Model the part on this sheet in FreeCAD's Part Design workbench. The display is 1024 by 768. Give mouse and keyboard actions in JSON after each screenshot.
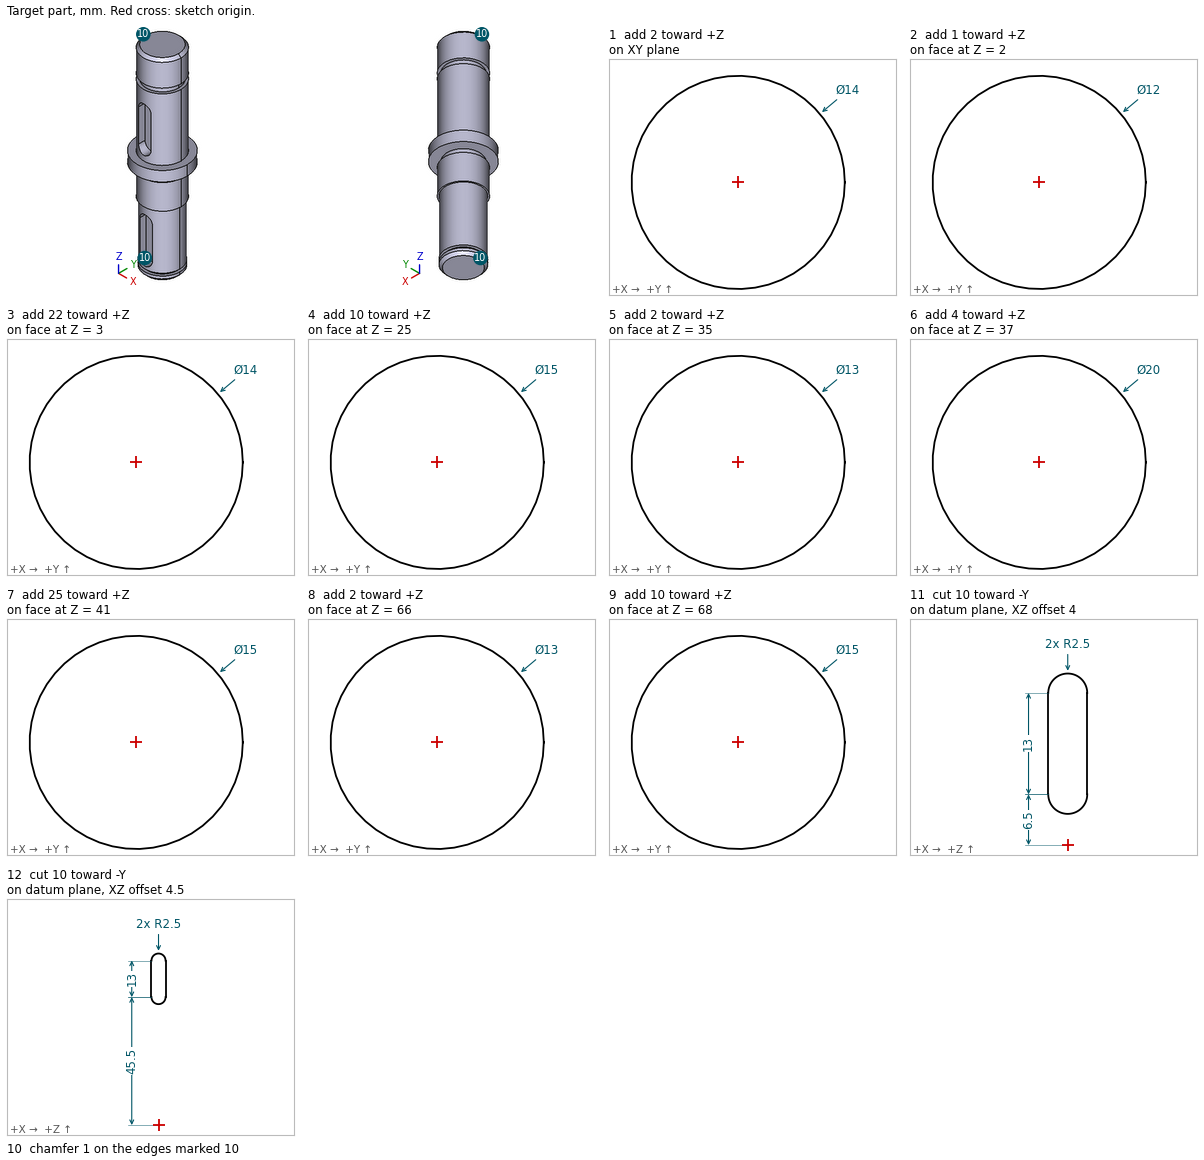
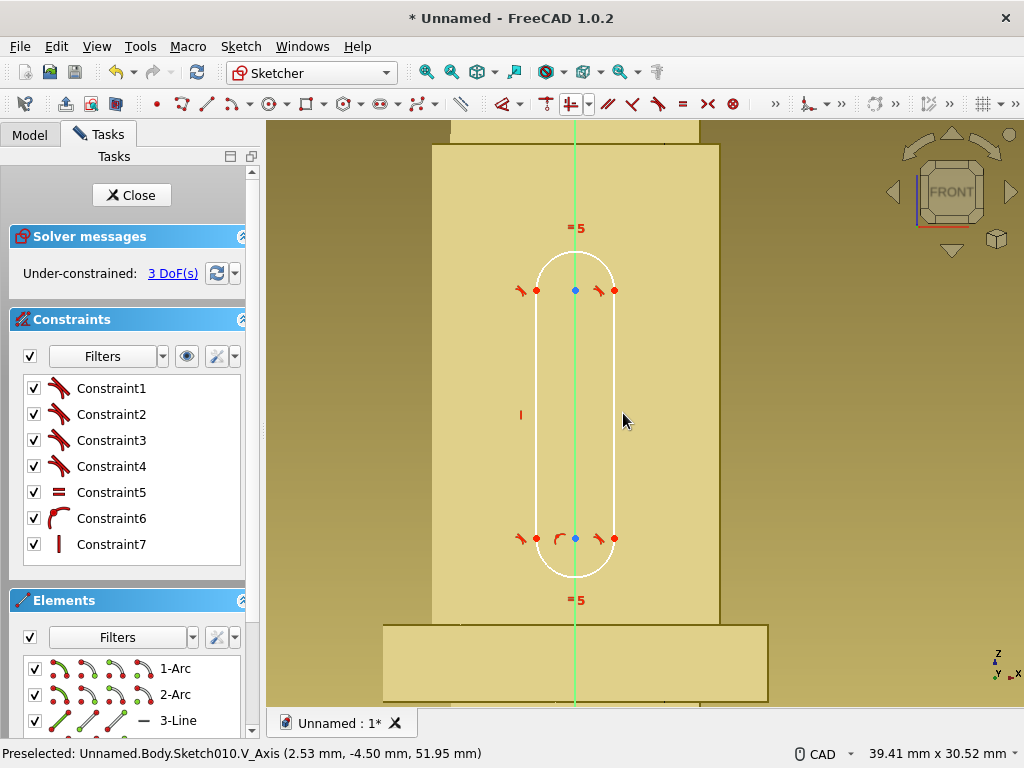
{"action": "left_click", "coordinate": [502, 104]}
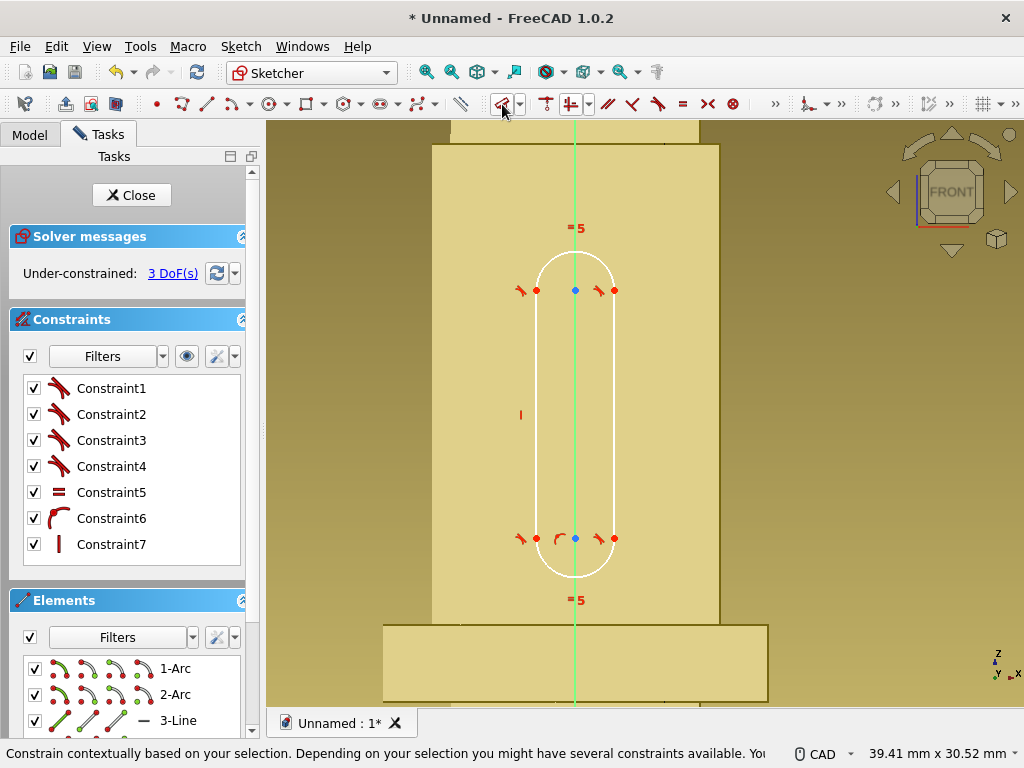
{"action": "left_click", "coordinate": [552, 570]}
{"action": "left_click", "coordinate": [533, 596]}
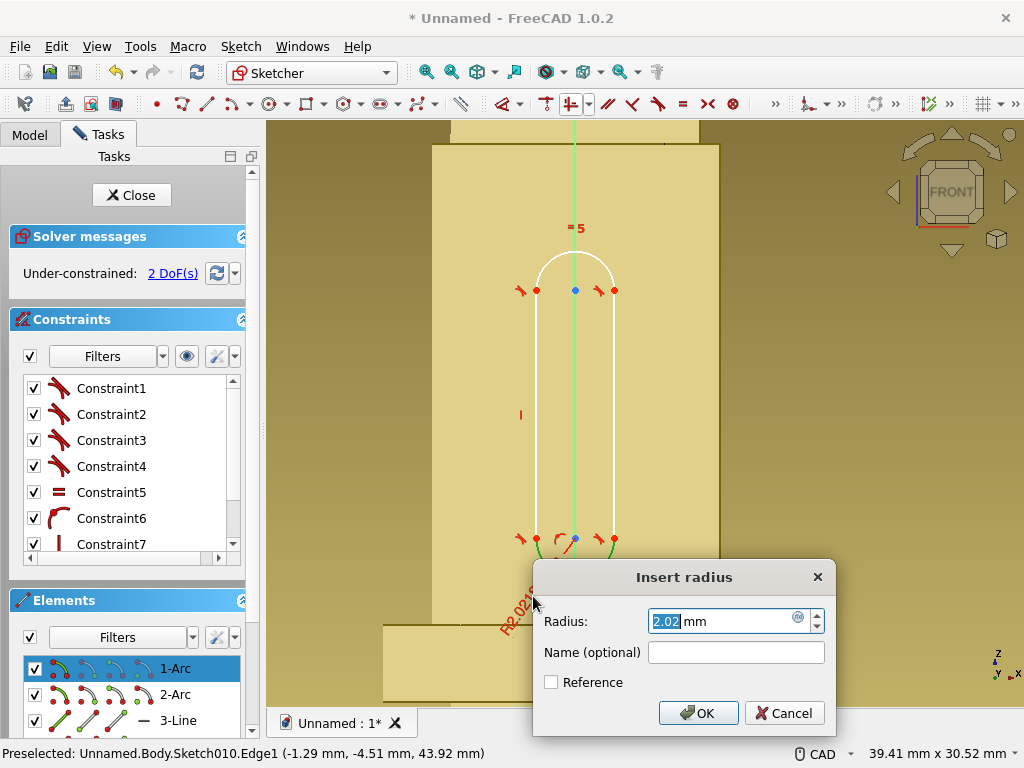
{"action": "type", "text": "2.5"}
{"action": "key", "text": "Return"}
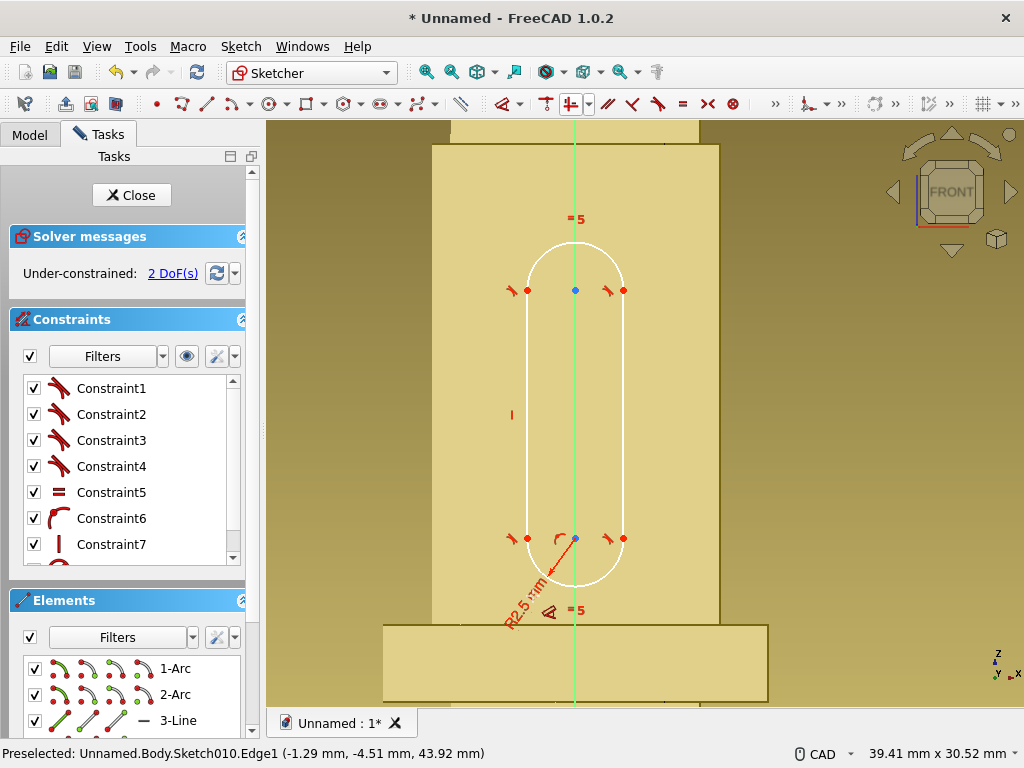
{"action": "left_click", "coordinate": [527, 464]}
{"action": "left_click", "coordinate": [493, 415]}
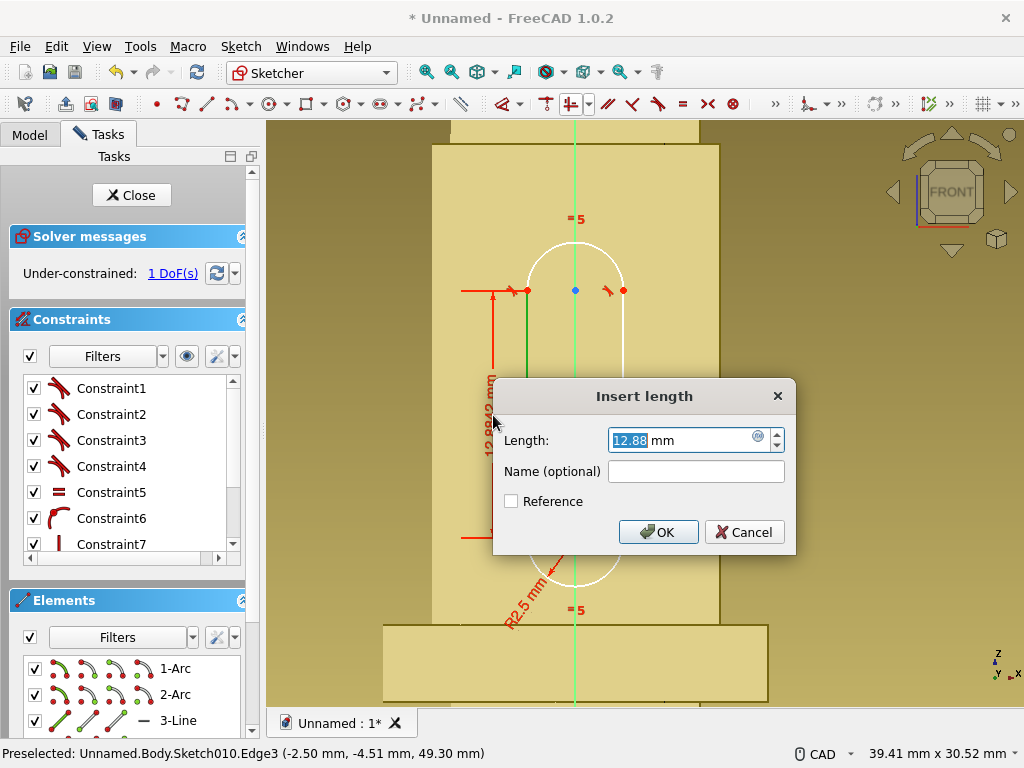
{"action": "type", "text": "13"}
{"action": "key", "text": "Return"}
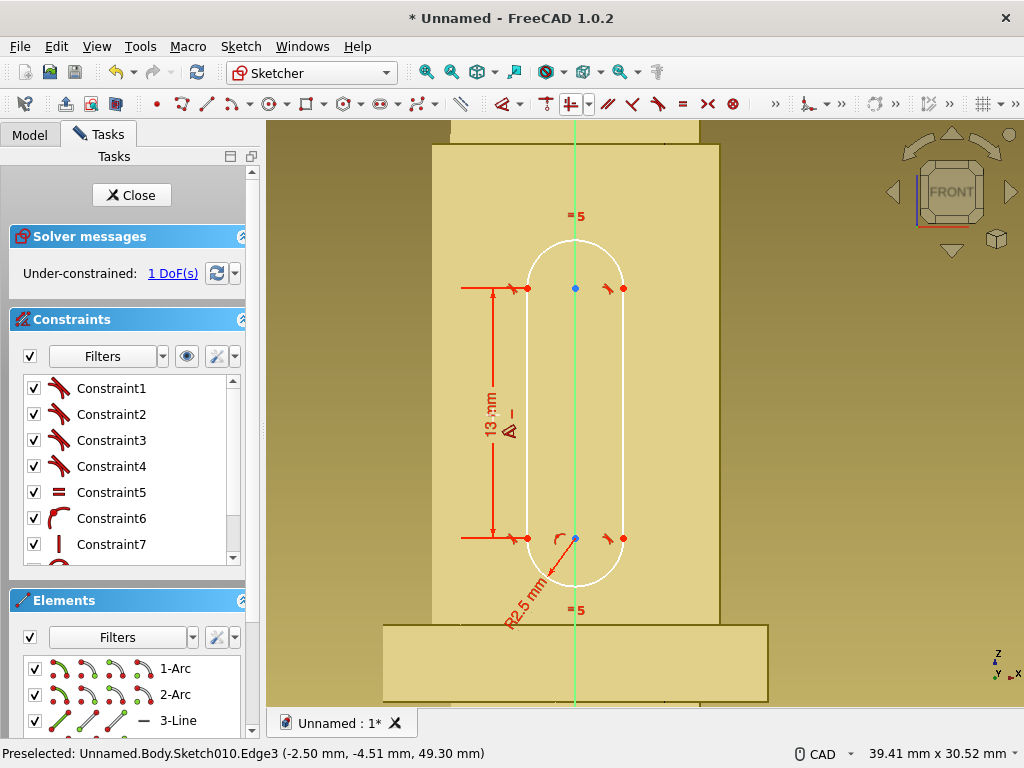
{"action": "left_click", "coordinate": [527, 538]}
{"action": "left_click", "coordinate": [493, 641]}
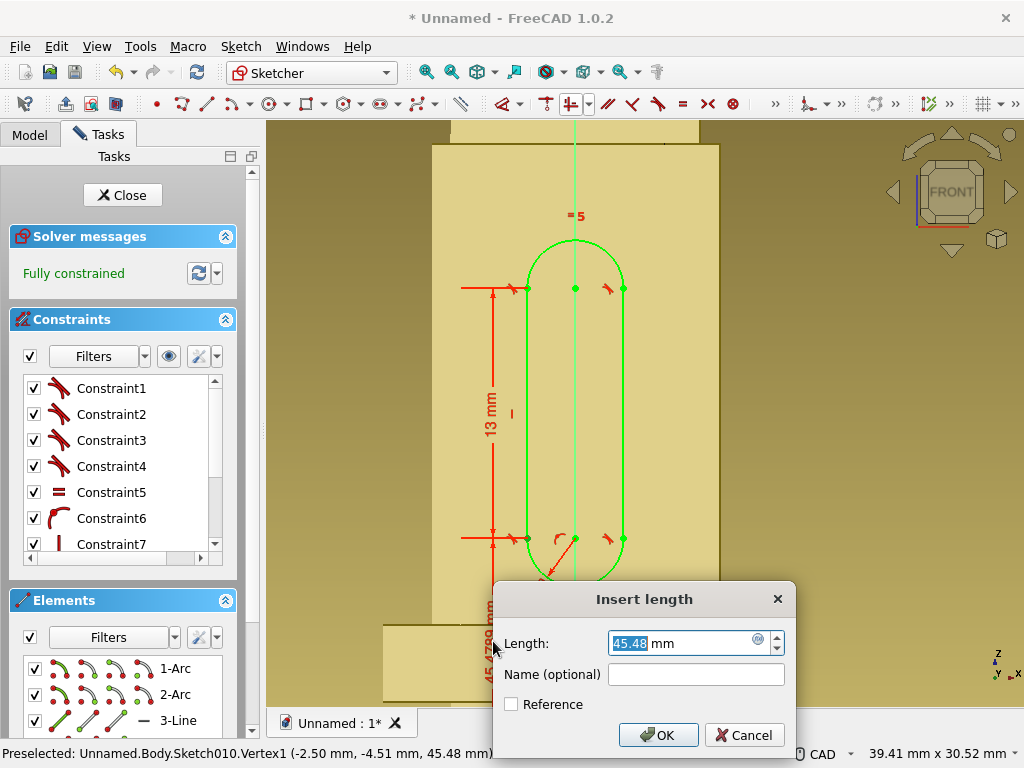
{"action": "type", "text": "45.5"}
{"action": "key", "text": "Return"}
{"action": "key", "text": "Escape"}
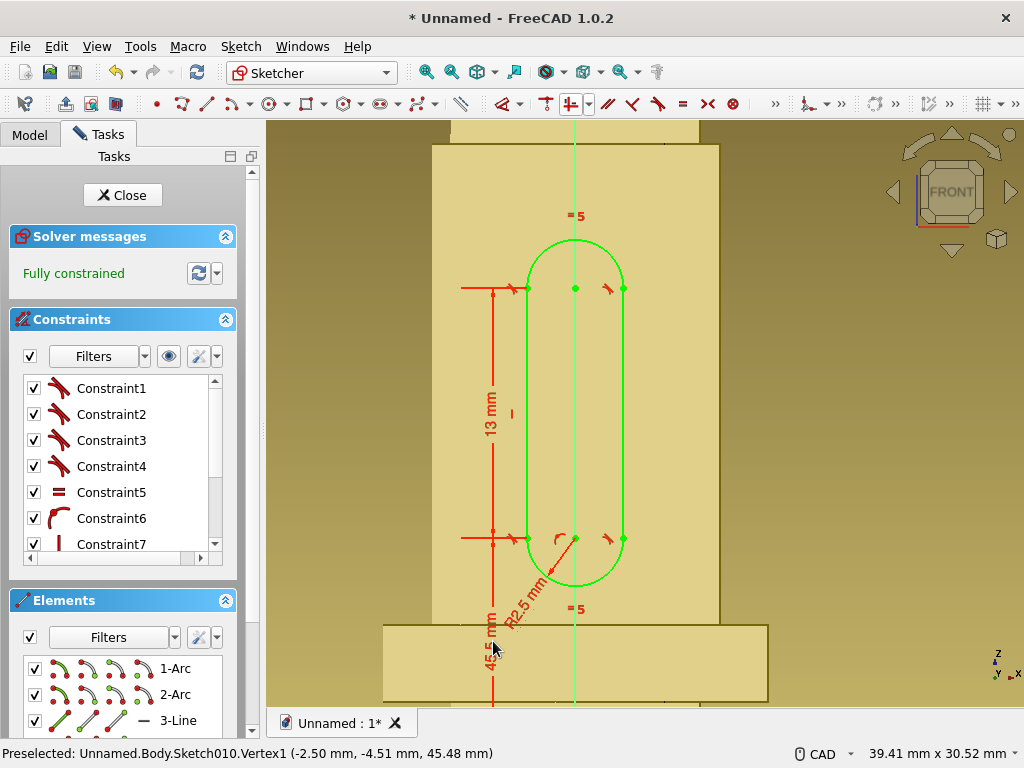
{"action": "left_click", "coordinate": [123, 195]}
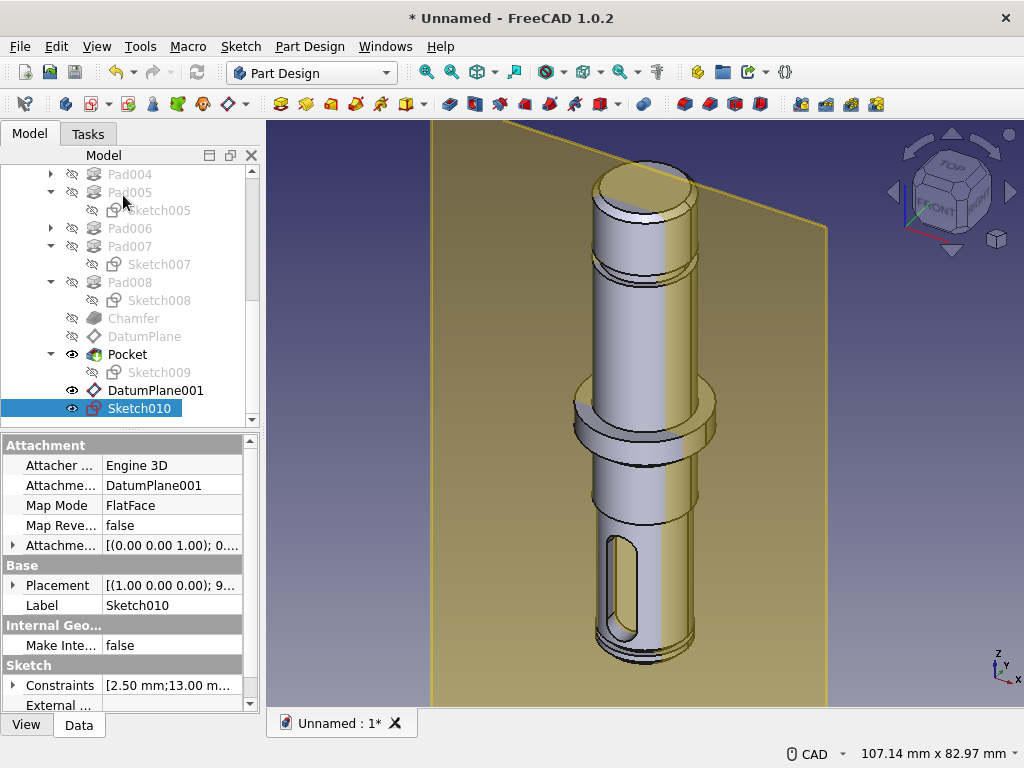
{"action": "left_click", "coordinate": [450, 104]}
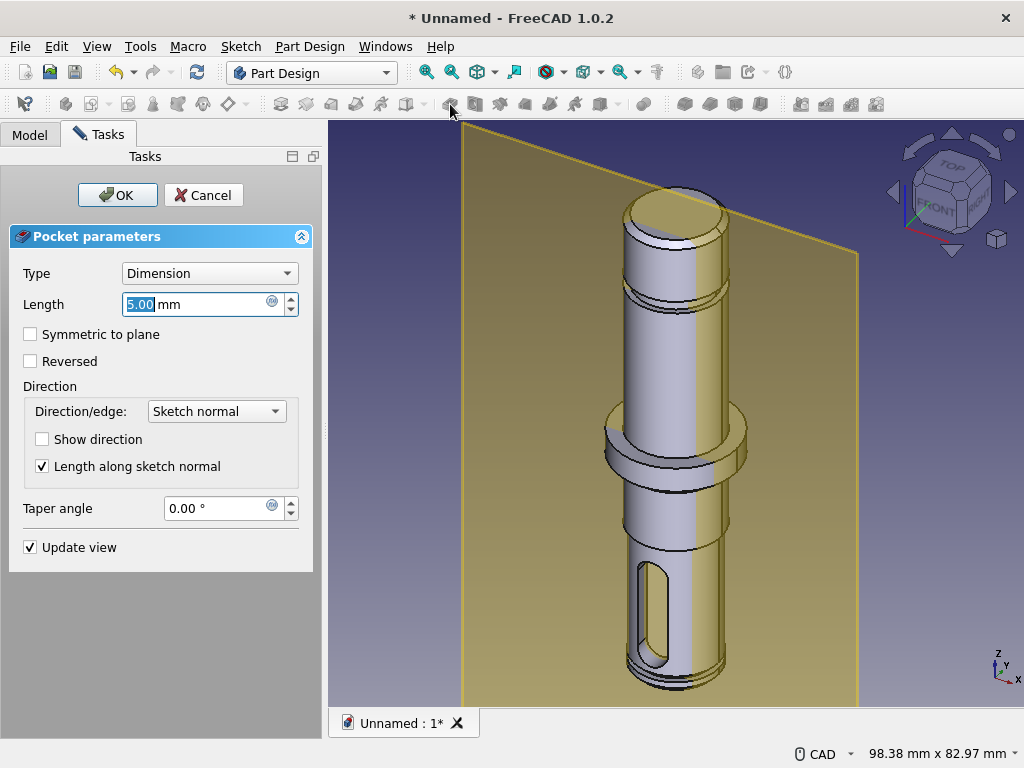
{"action": "type", "text": "10"}
{"action": "key", "text": "Tab"}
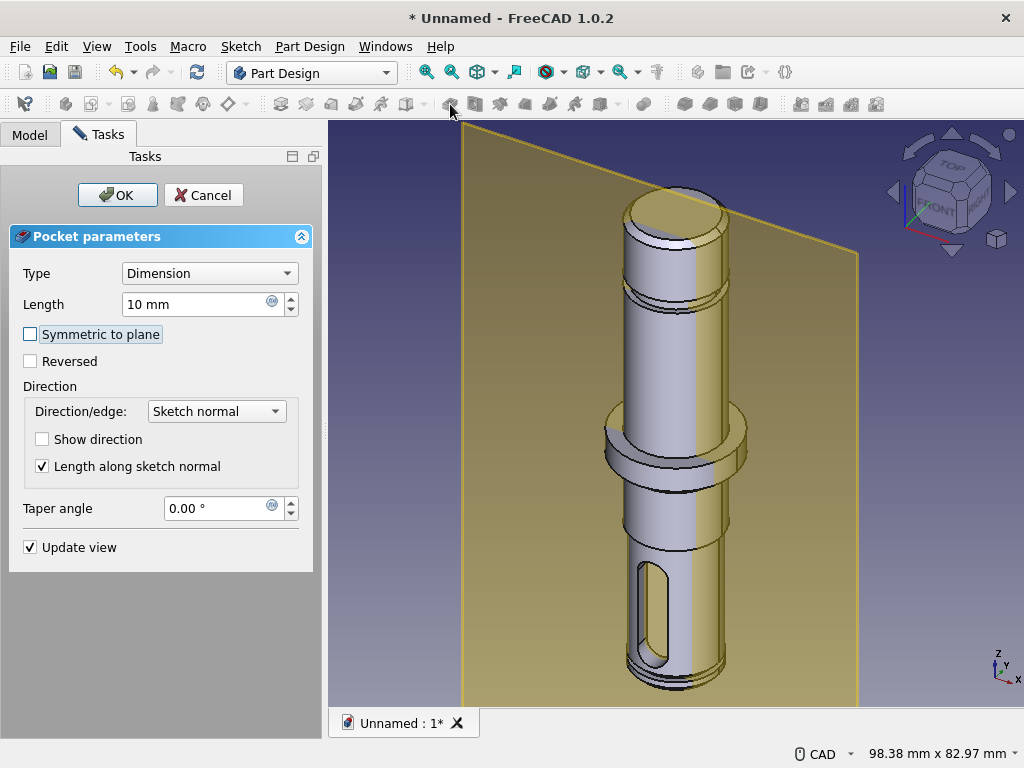
{"action": "left_click", "coordinate": [31, 361]}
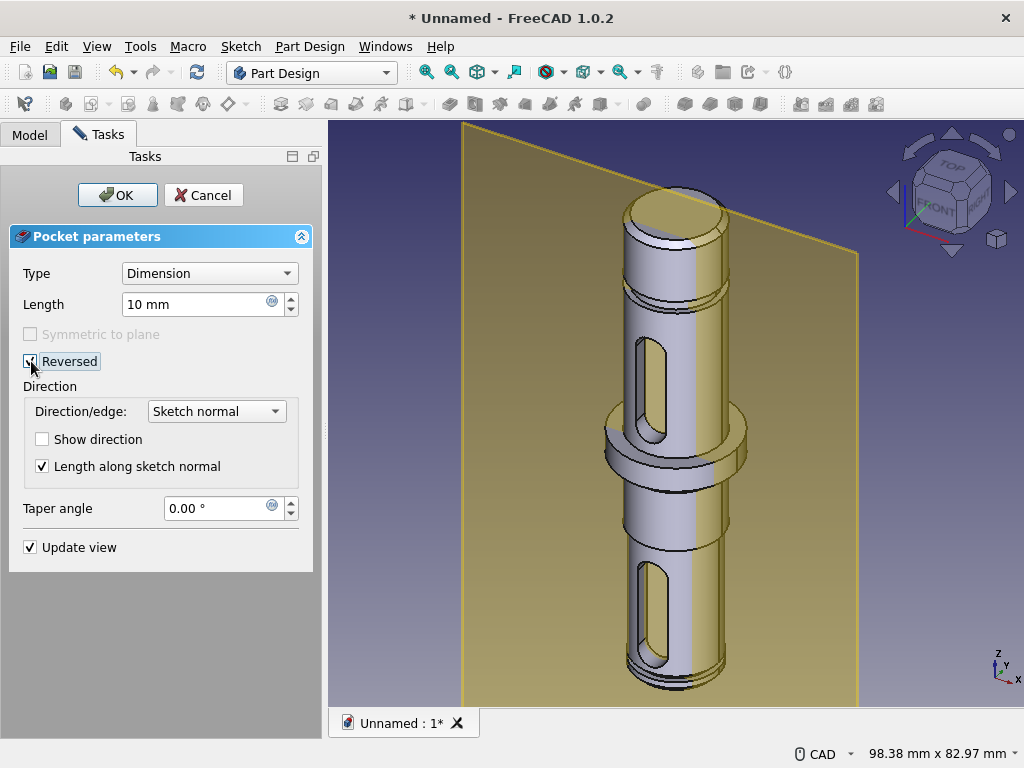
{"action": "left_click", "coordinate": [118, 195]}